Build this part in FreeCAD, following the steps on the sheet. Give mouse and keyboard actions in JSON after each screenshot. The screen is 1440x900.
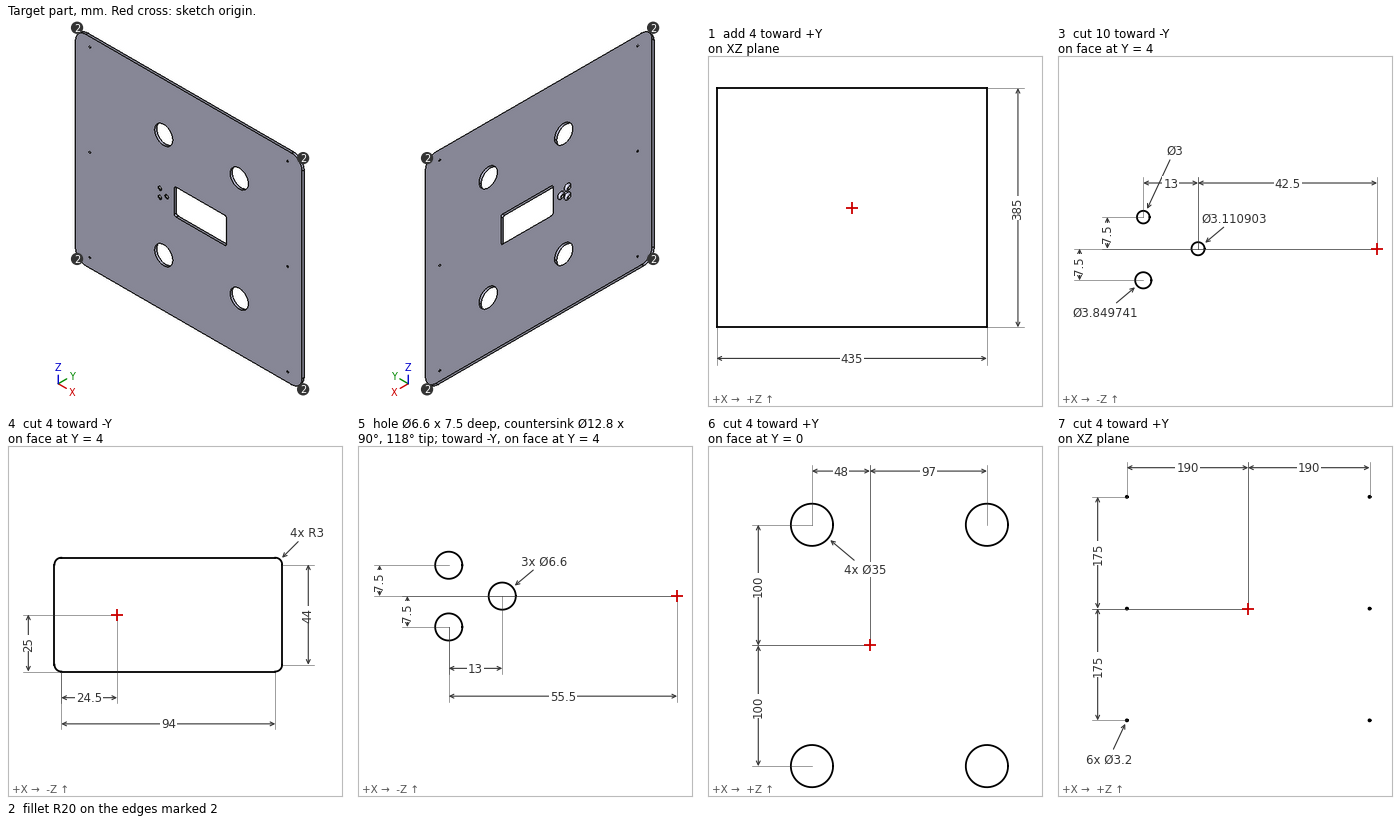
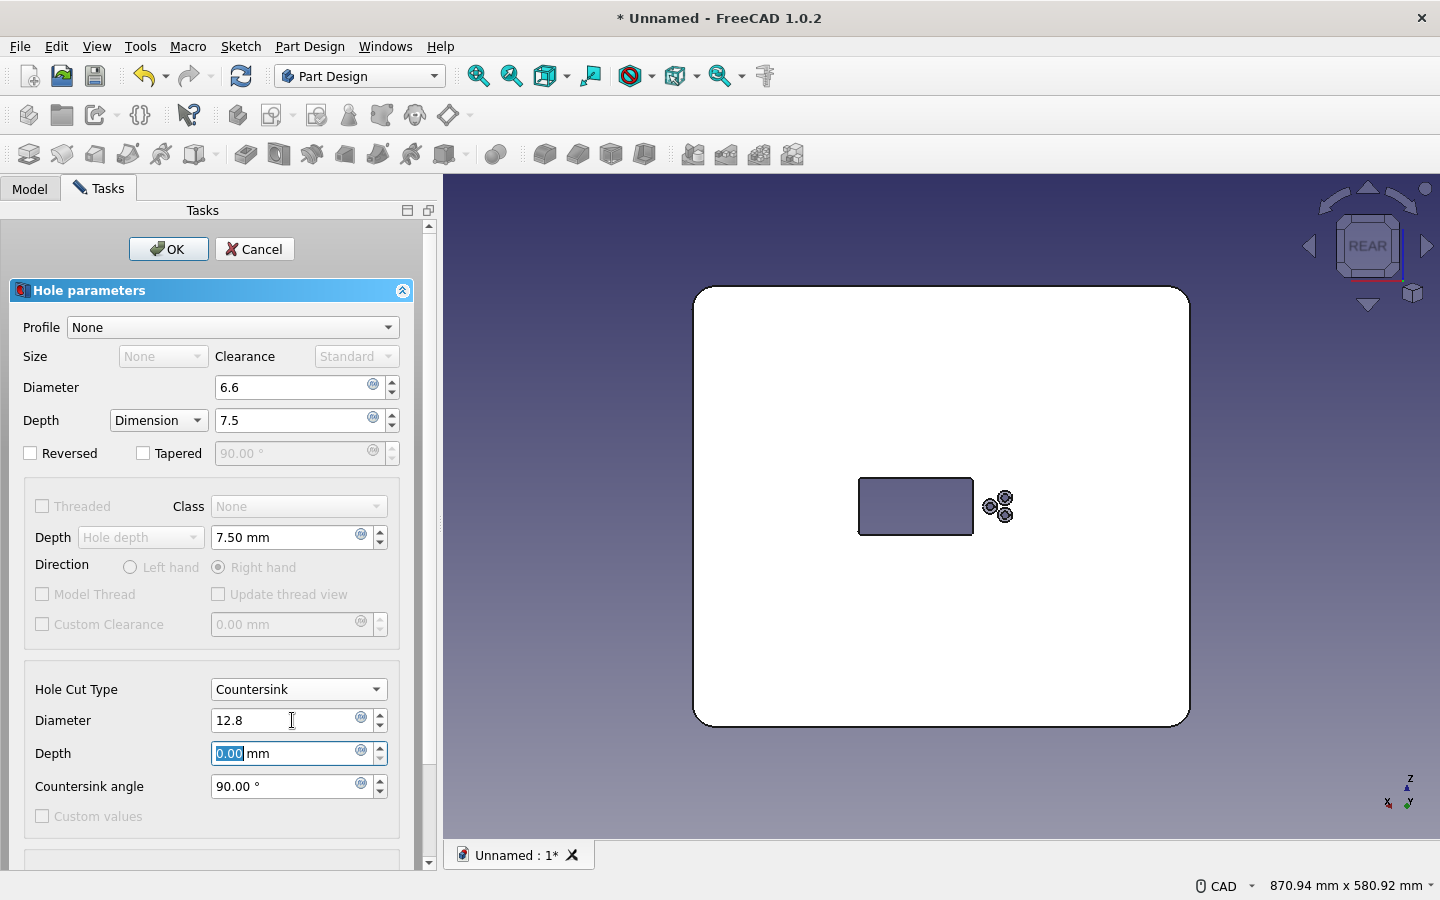
{"action": "left_click", "coordinate": [169, 249]}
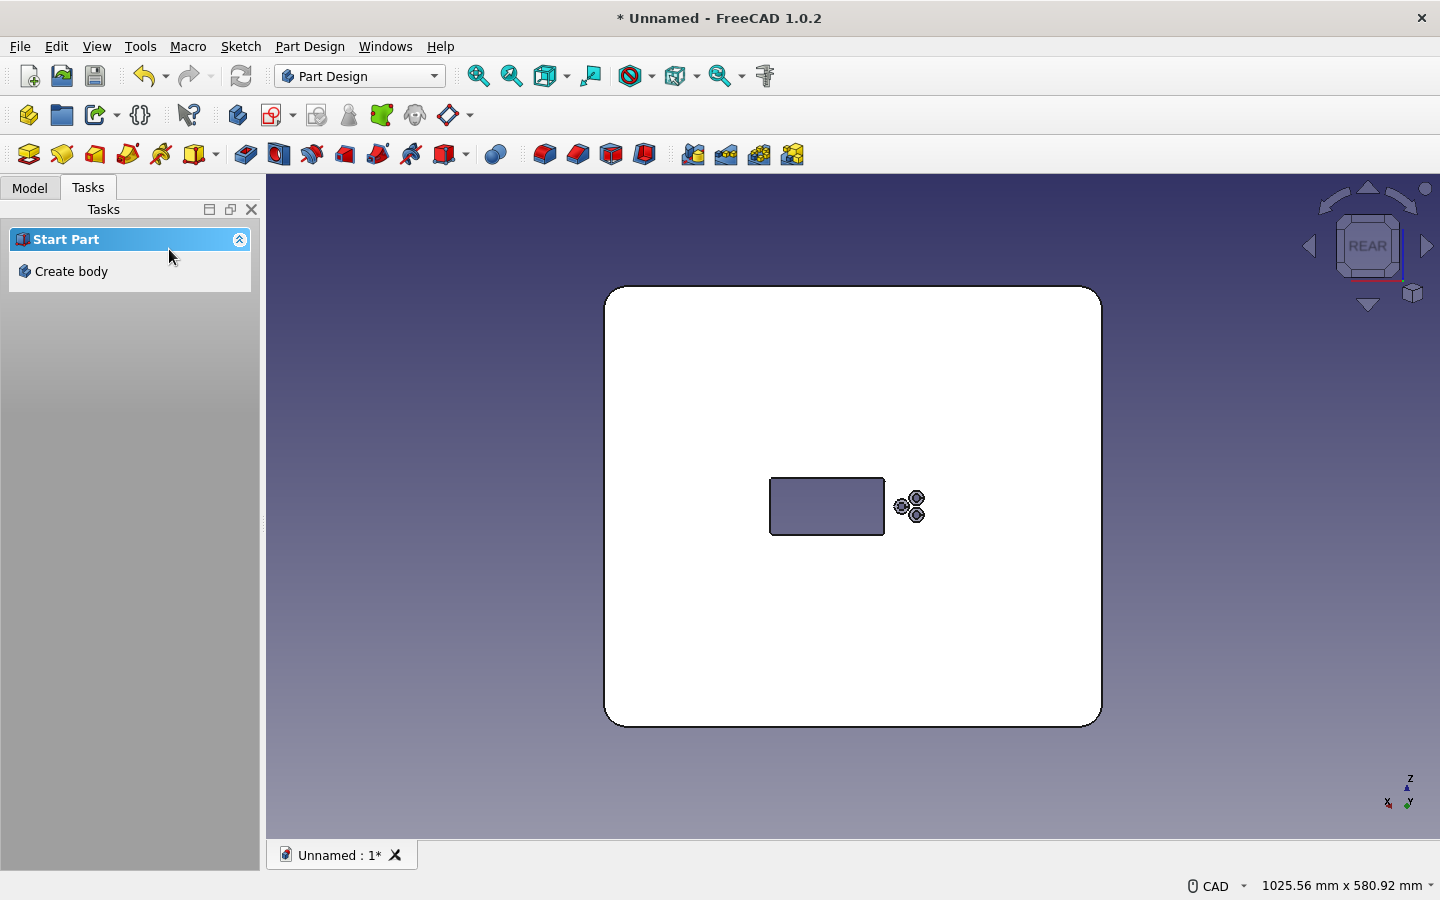
{"action": "key", "text": "0"}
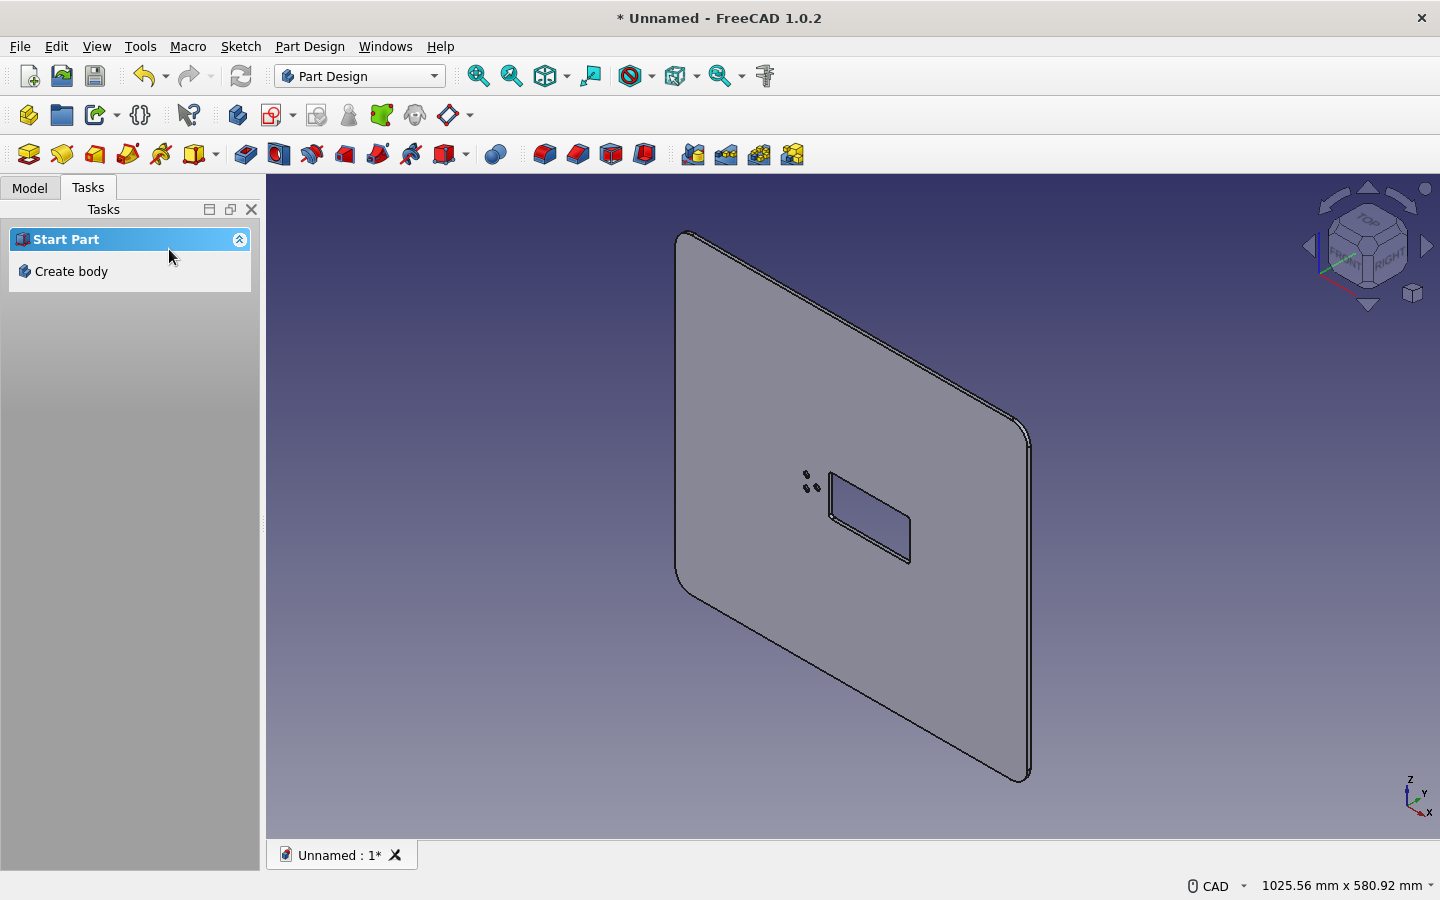
{"action": "left_click", "coordinate": [952, 462]}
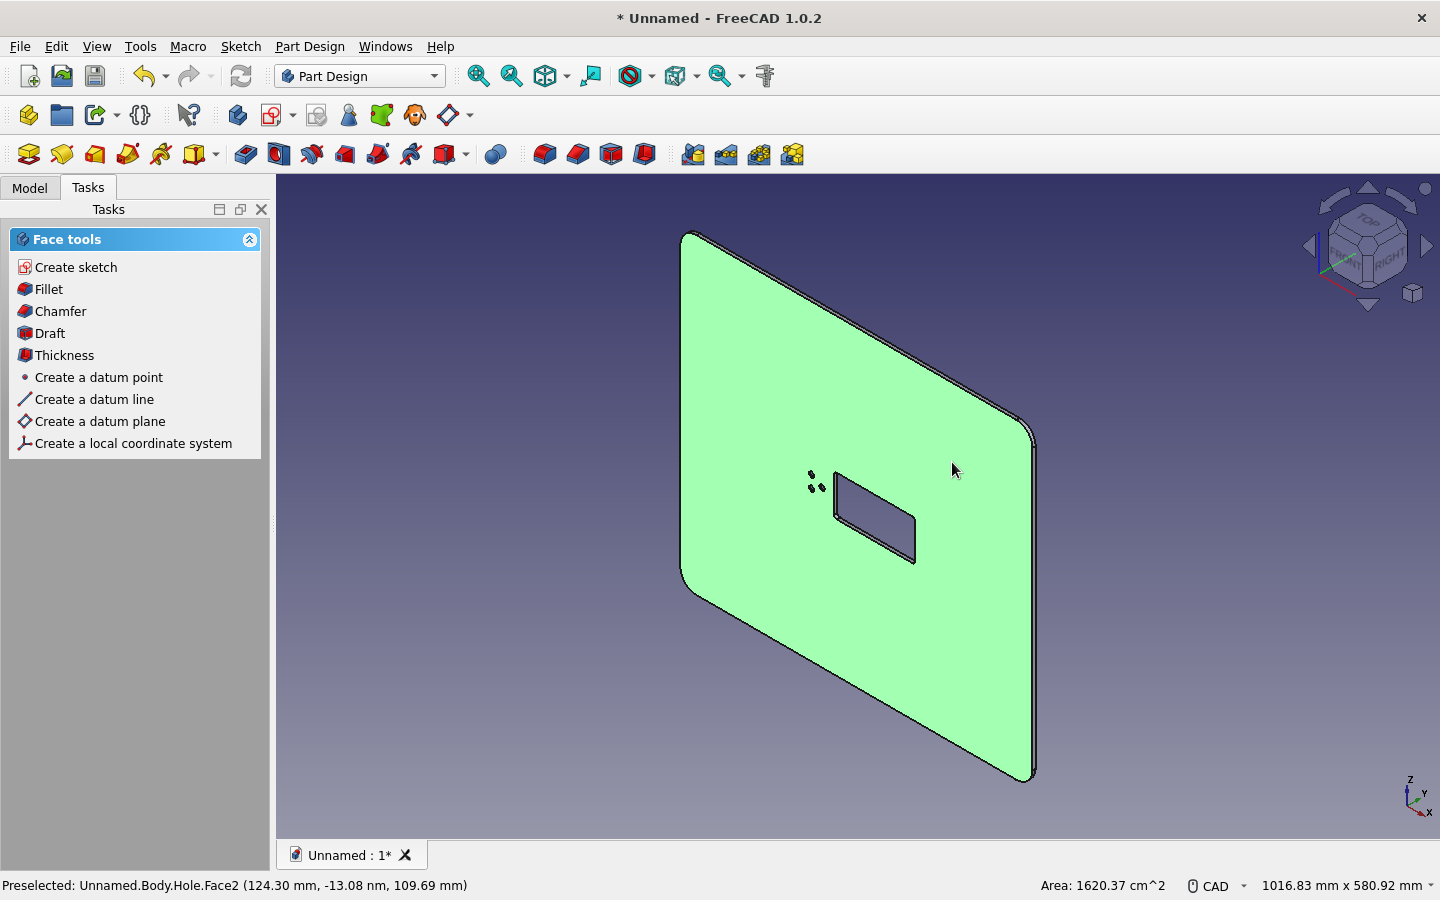
{"action": "left_click", "coordinate": [270, 116]}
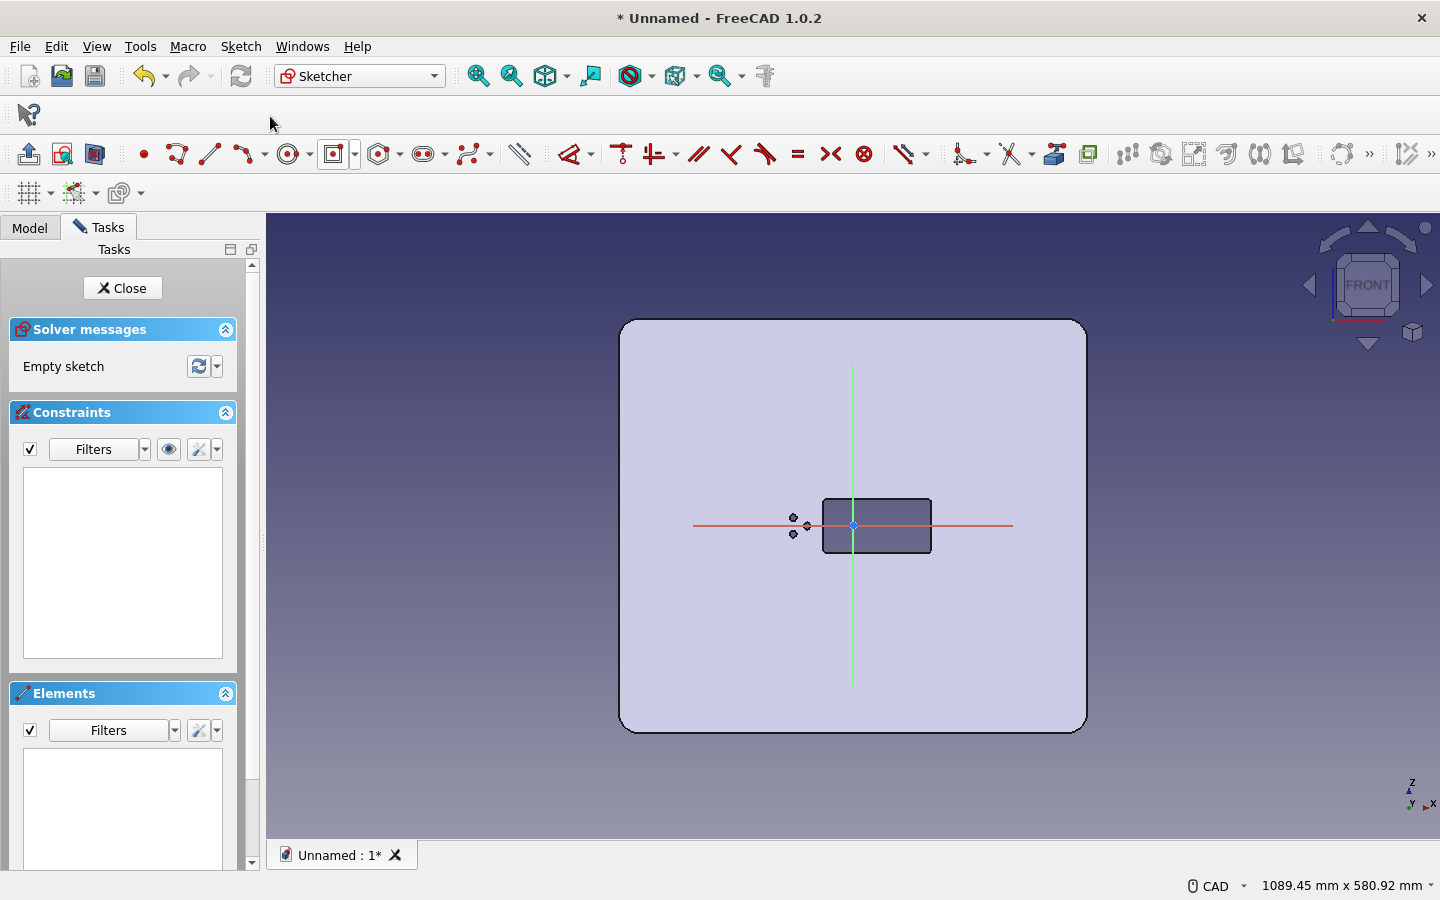
{"action": "scroll", "coordinate": [1072, 526], "scroll_direction": "up", "scroll_amount": 2}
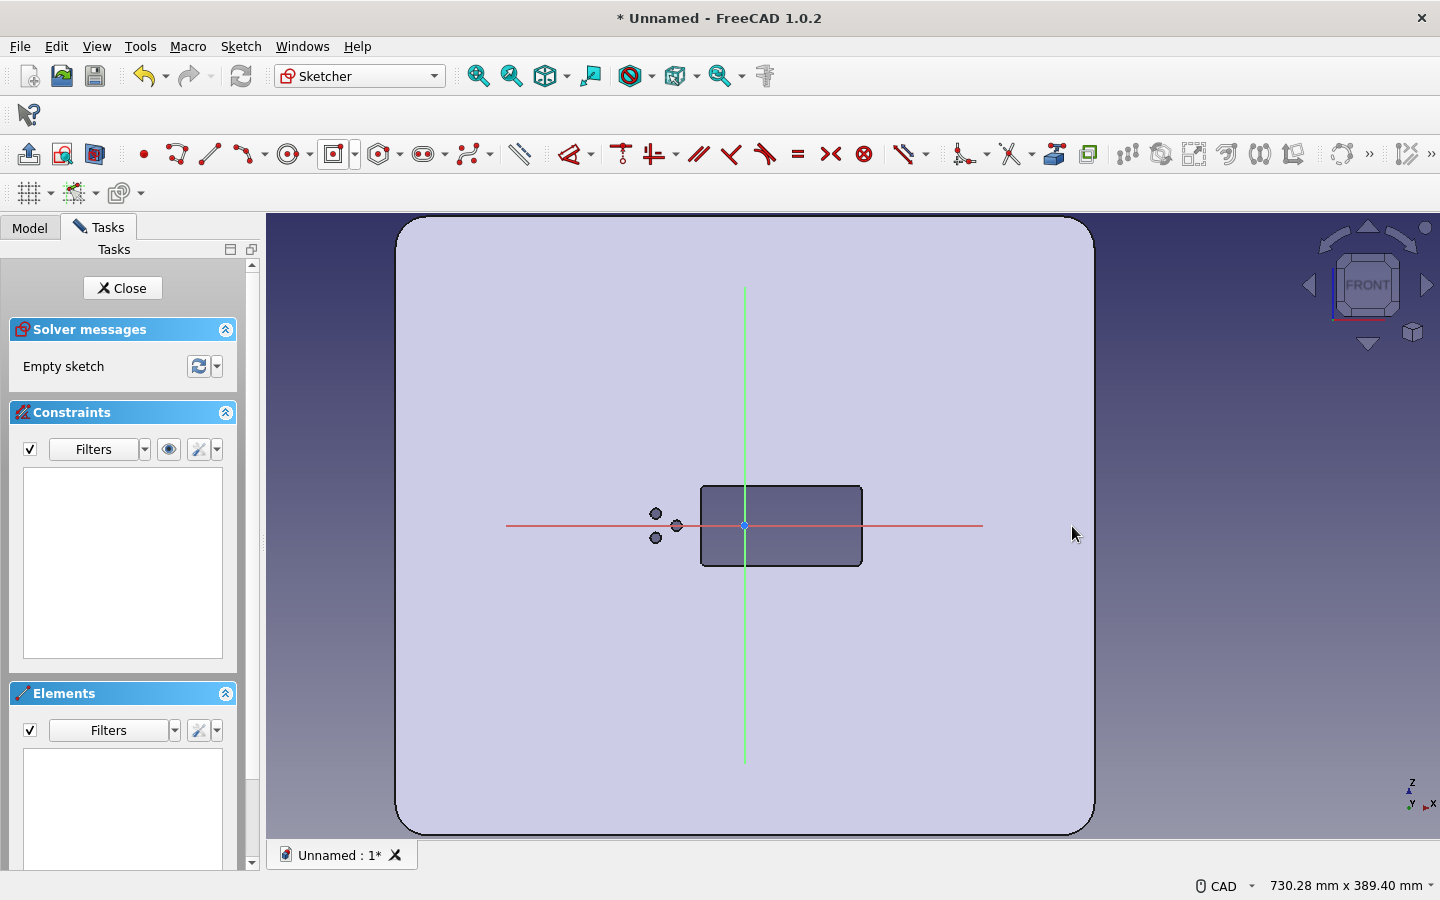
{"action": "left_click", "coordinate": [288, 154]}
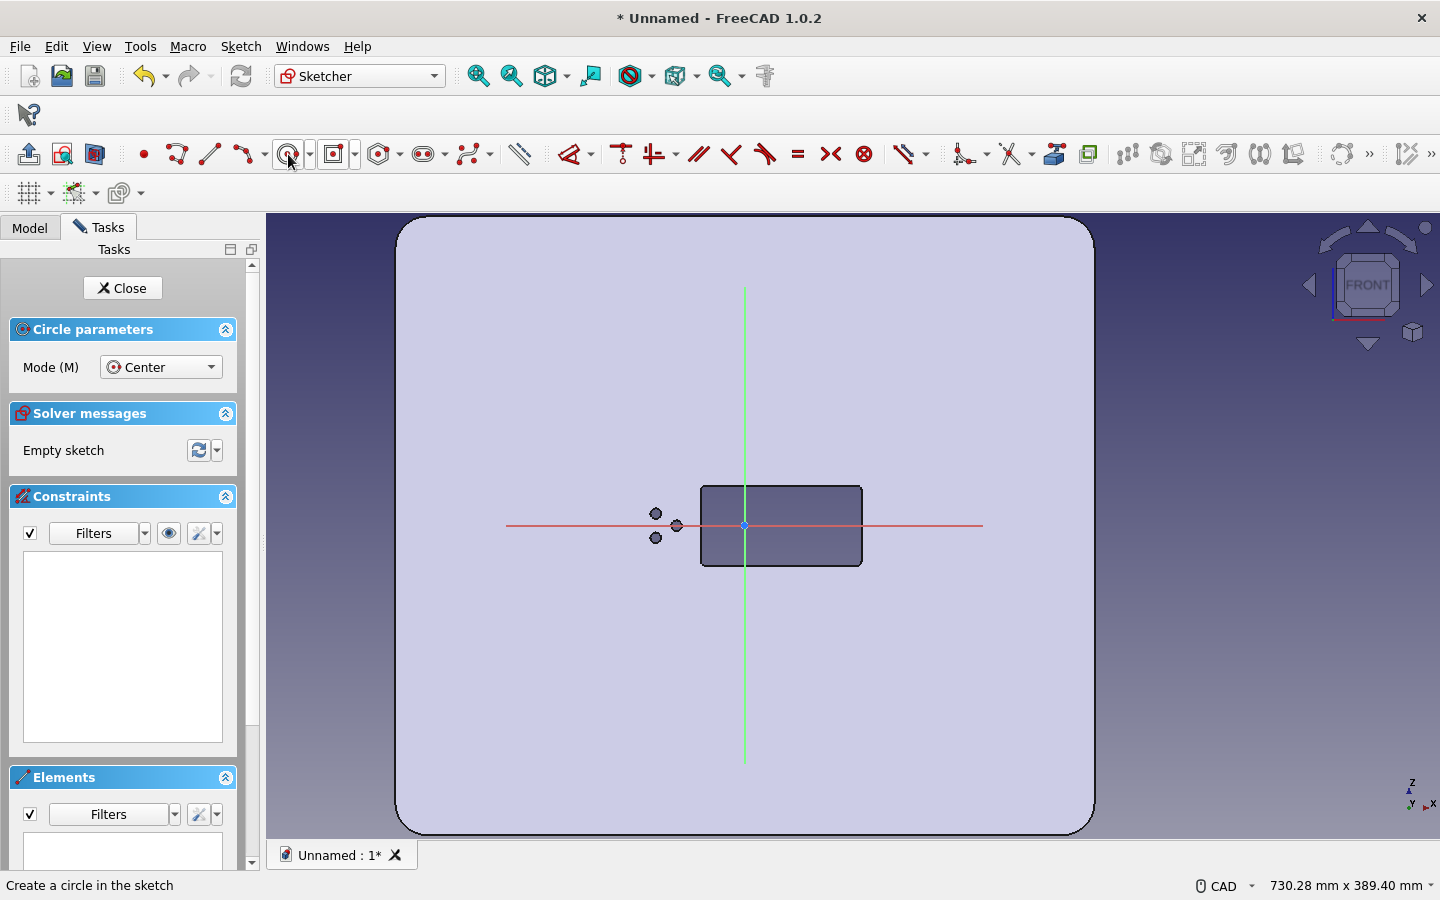
{"action": "left_click", "coordinate": [668, 365]}
{"action": "left_click", "coordinate": [688, 345]}